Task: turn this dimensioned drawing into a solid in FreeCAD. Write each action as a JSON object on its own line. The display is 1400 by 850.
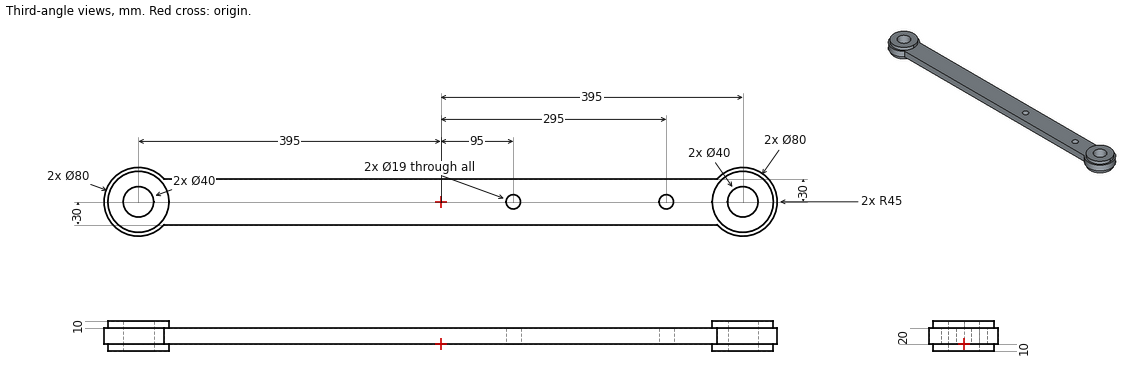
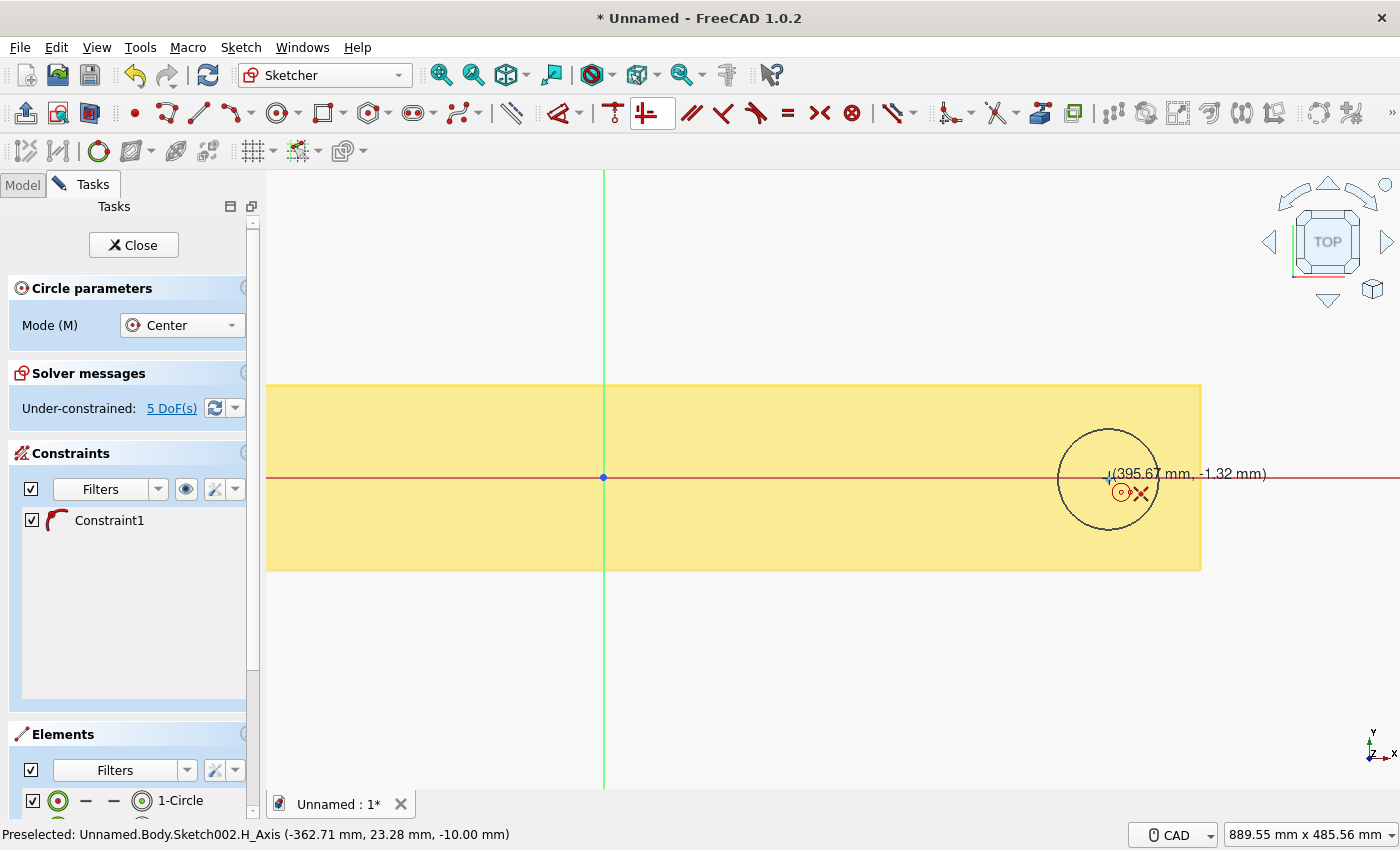
{"action": "left_click", "coordinate": [1108, 479]}
{"action": "left_click", "coordinate": [1126, 460]}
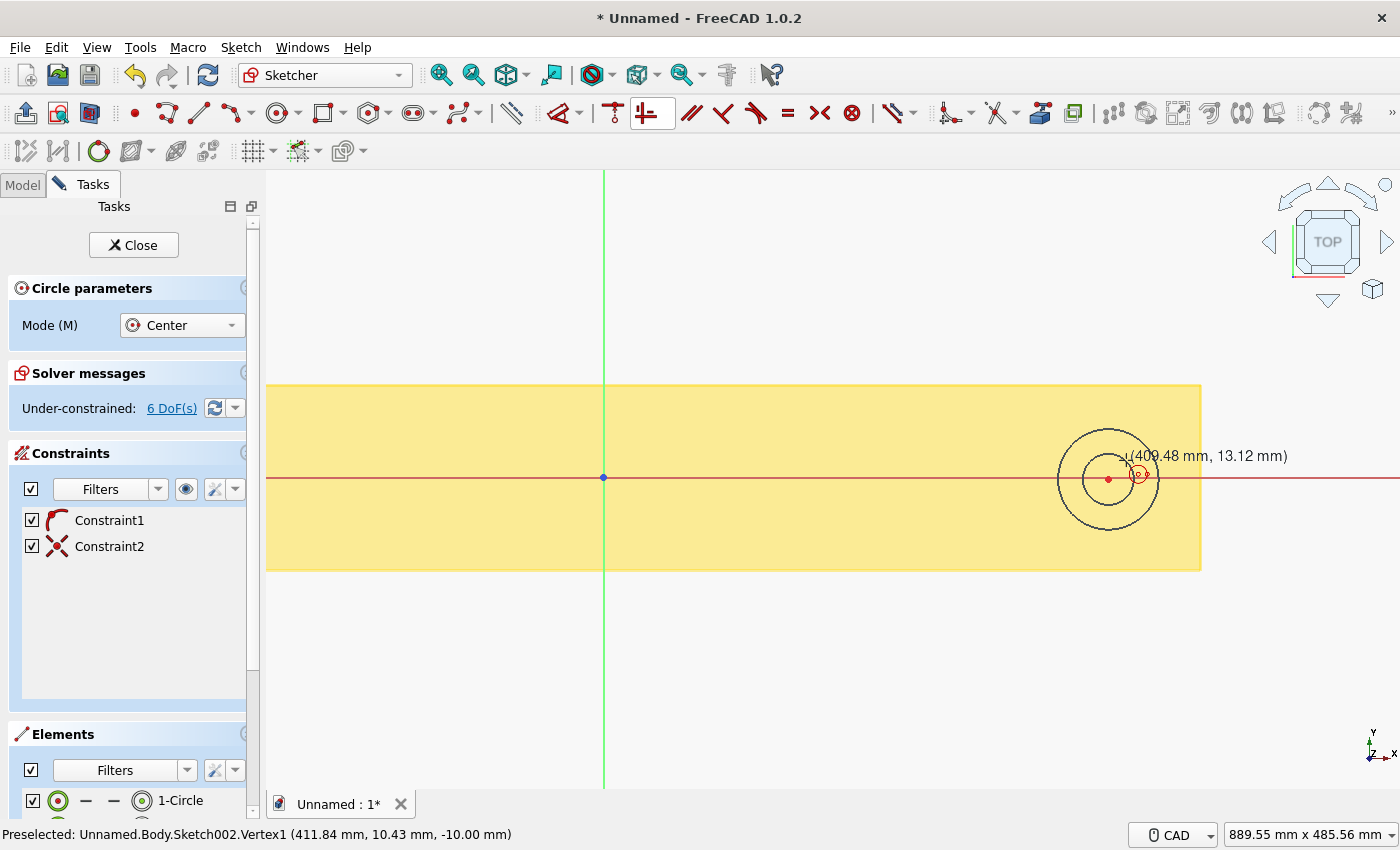
{"action": "scroll", "coordinate": [960, 482], "scroll_direction": "down", "scroll_amount": 3}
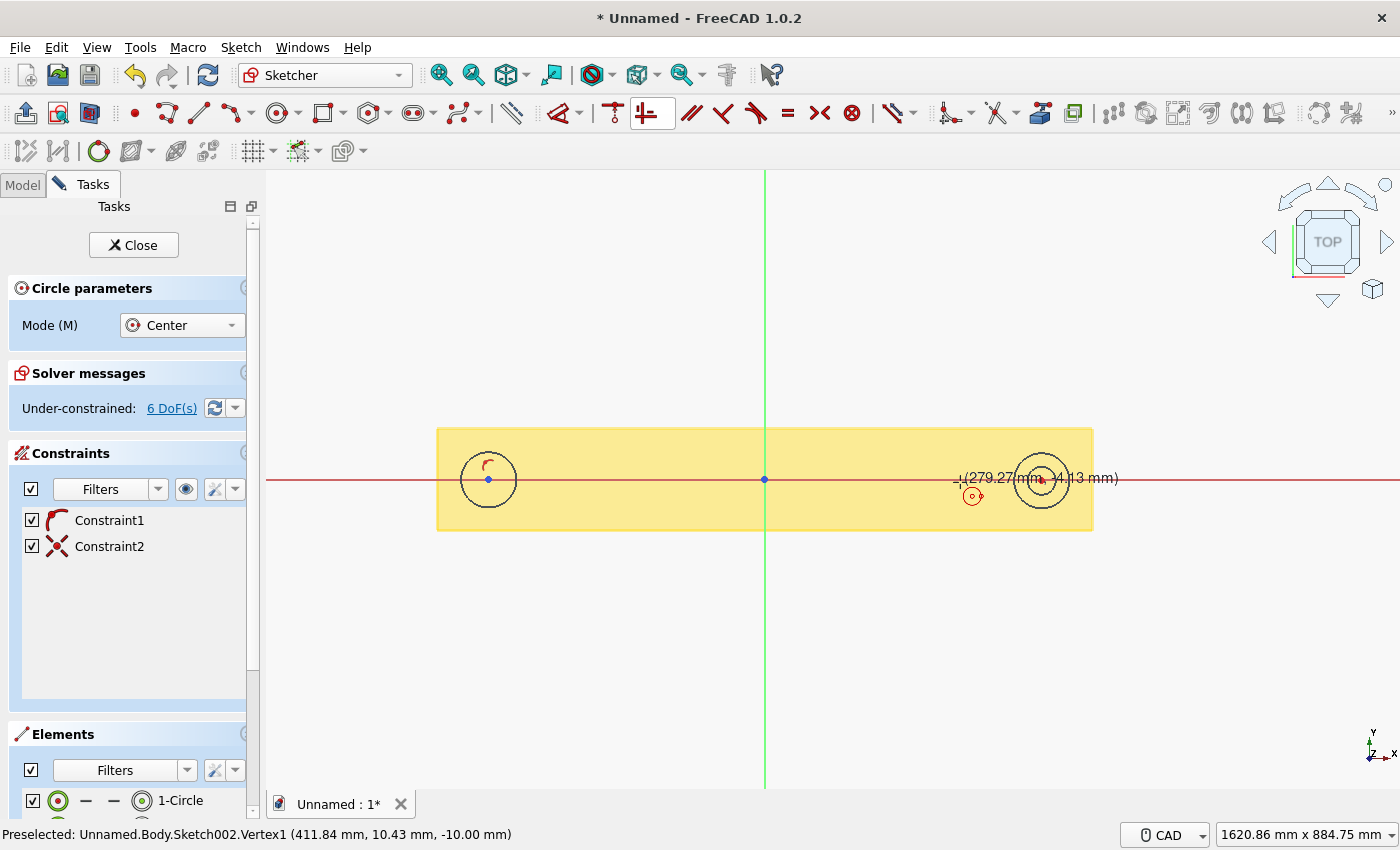
{"action": "scroll", "coordinate": [489, 480], "scroll_direction": "up", "scroll_amount": 3}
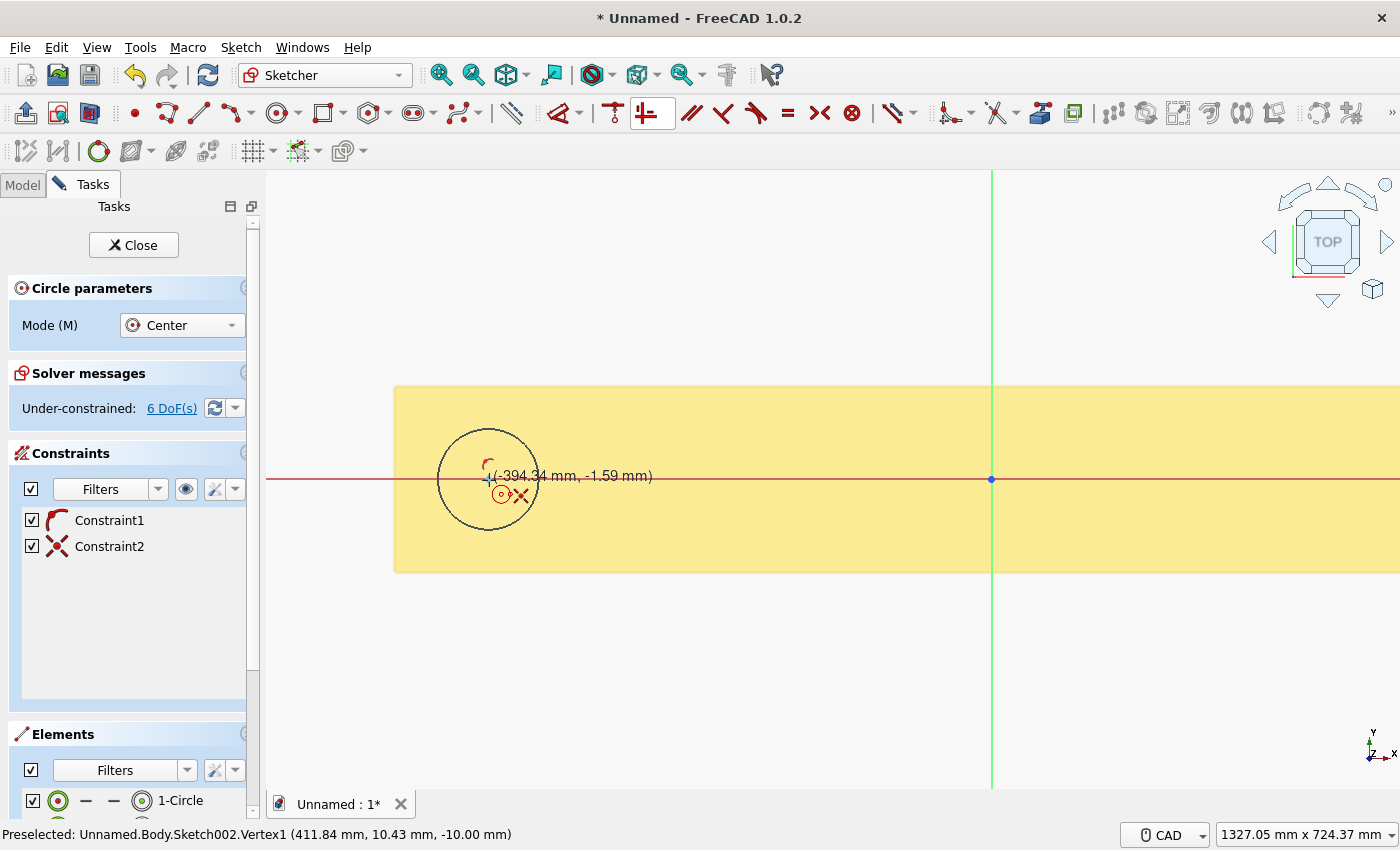
{"action": "left_click", "coordinate": [488, 479]}
{"action": "left_click", "coordinate": [506, 461]}
{"action": "key", "text": "Escape"}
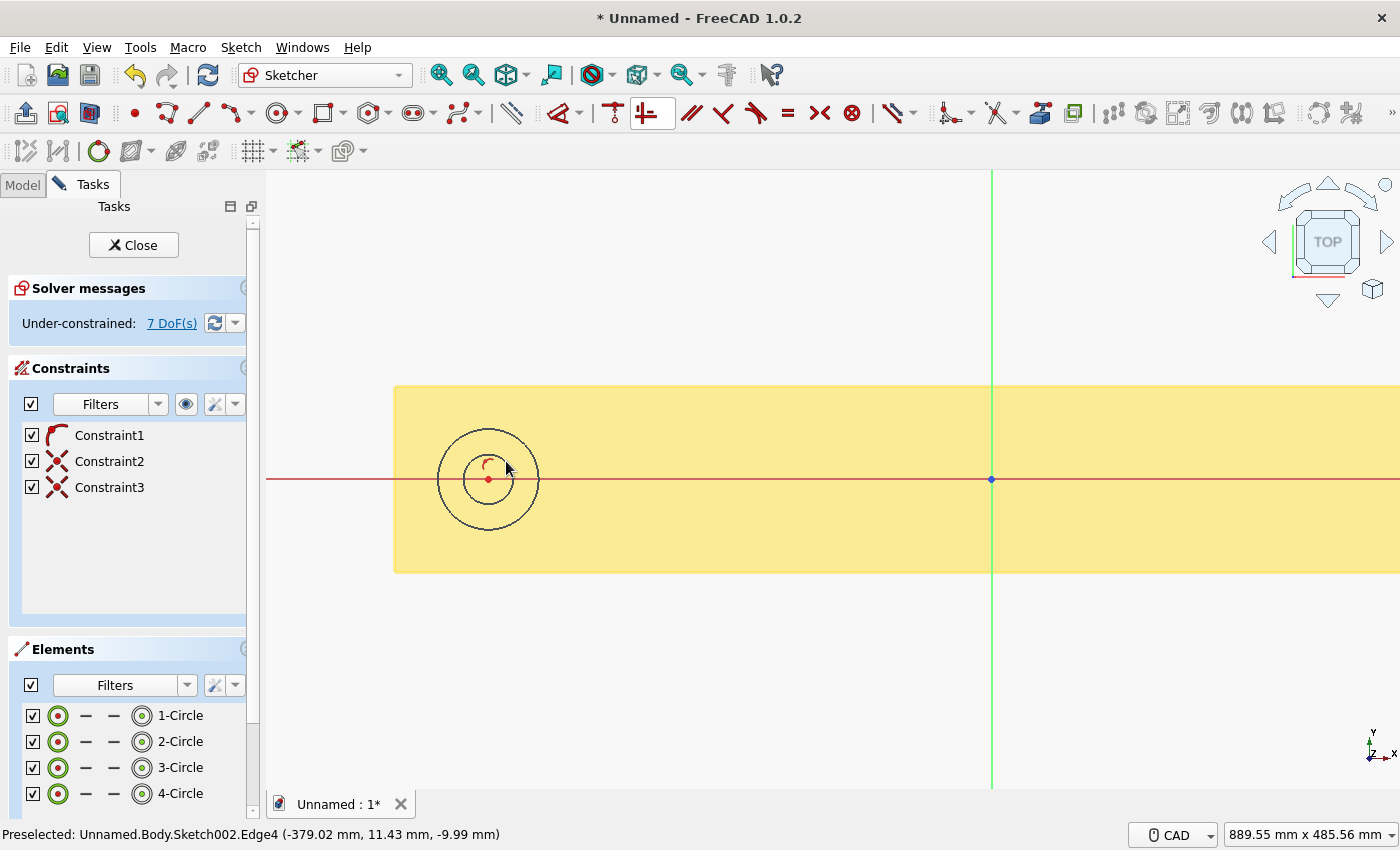
{"action": "scroll", "coordinate": [488, 480], "scroll_direction": "down", "scroll_amount": 3}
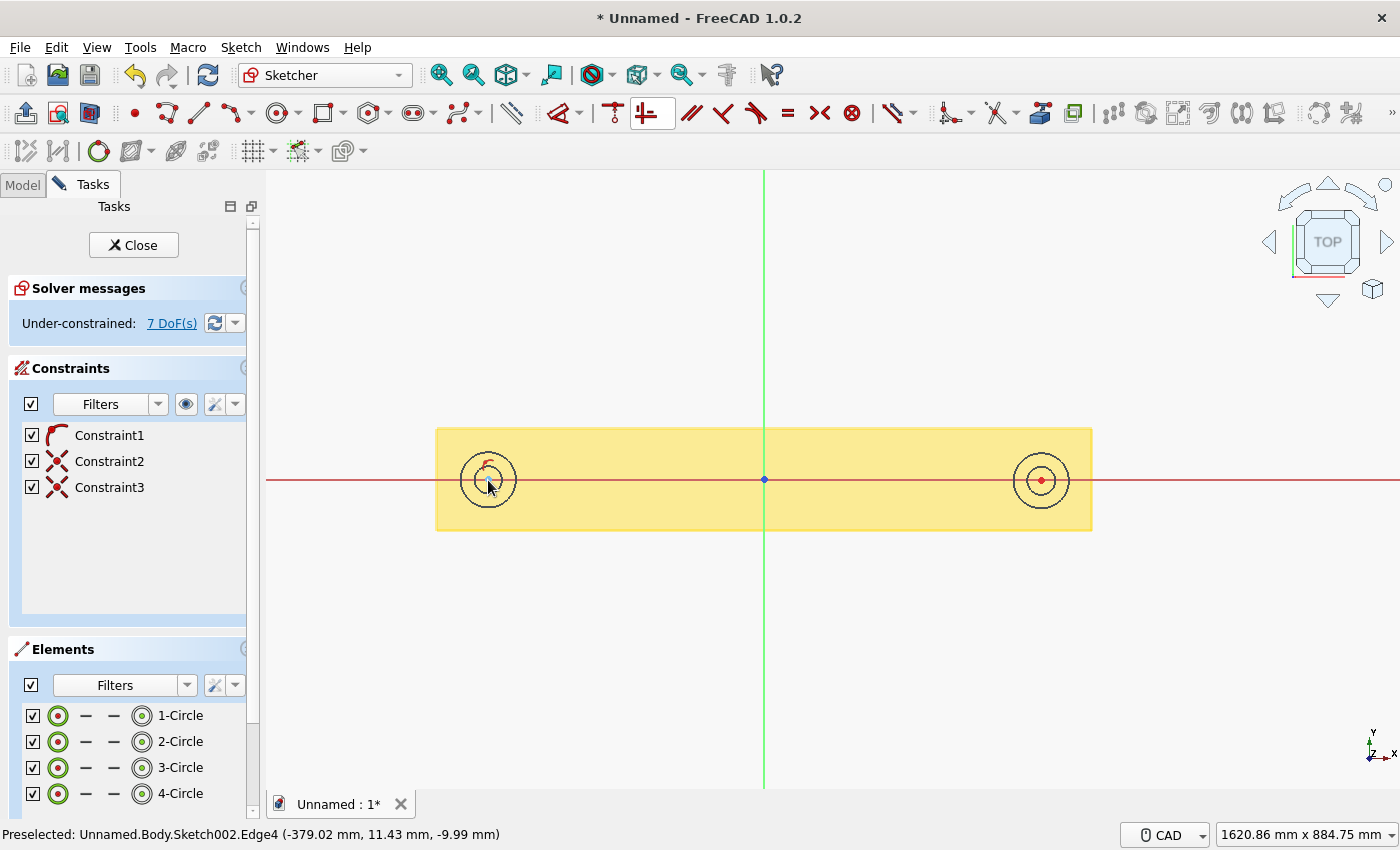
{"action": "left_click", "coordinate": [1061, 461]}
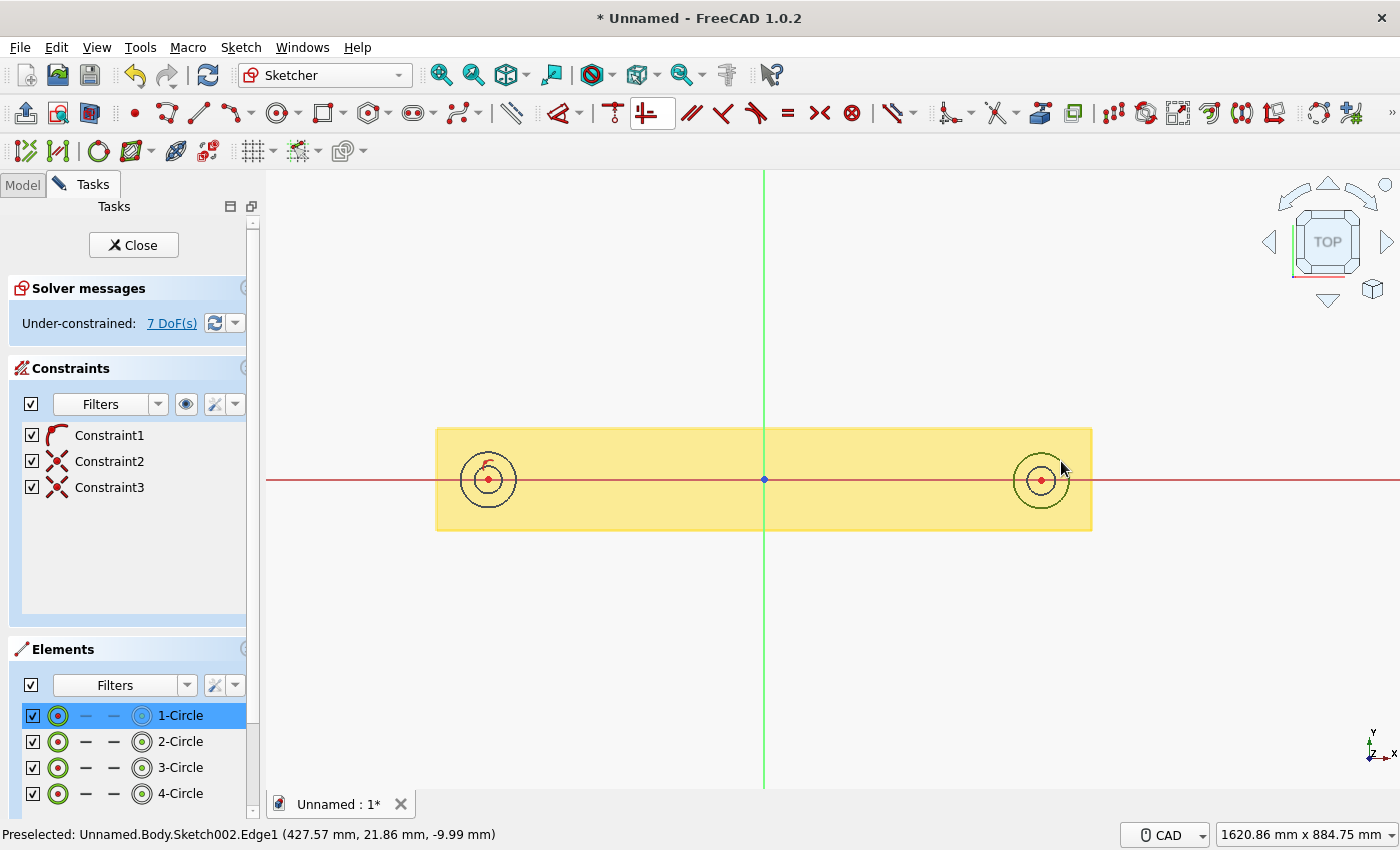
{"action": "left_click", "coordinate": [508, 460]}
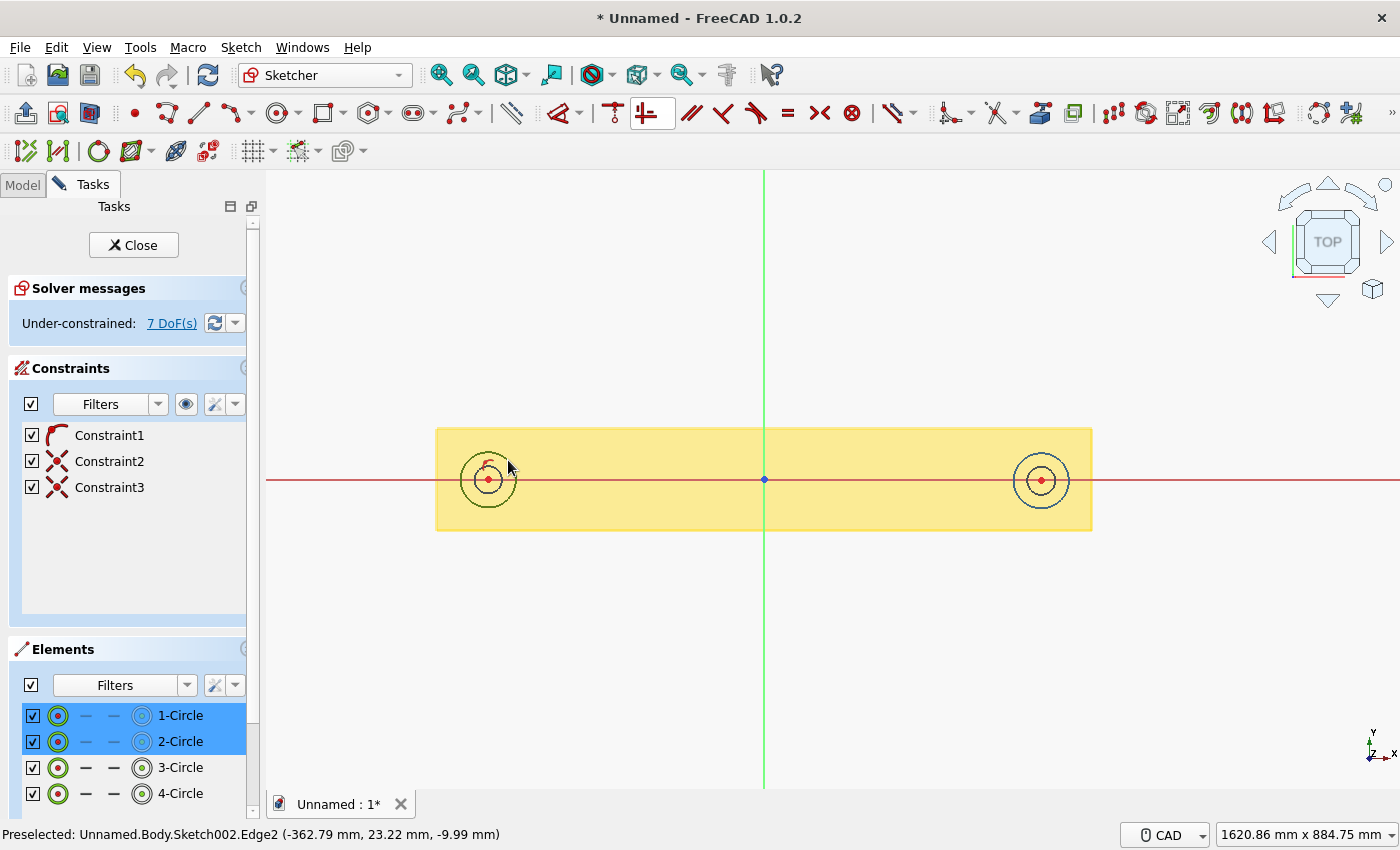
{"action": "key", "text": "e"}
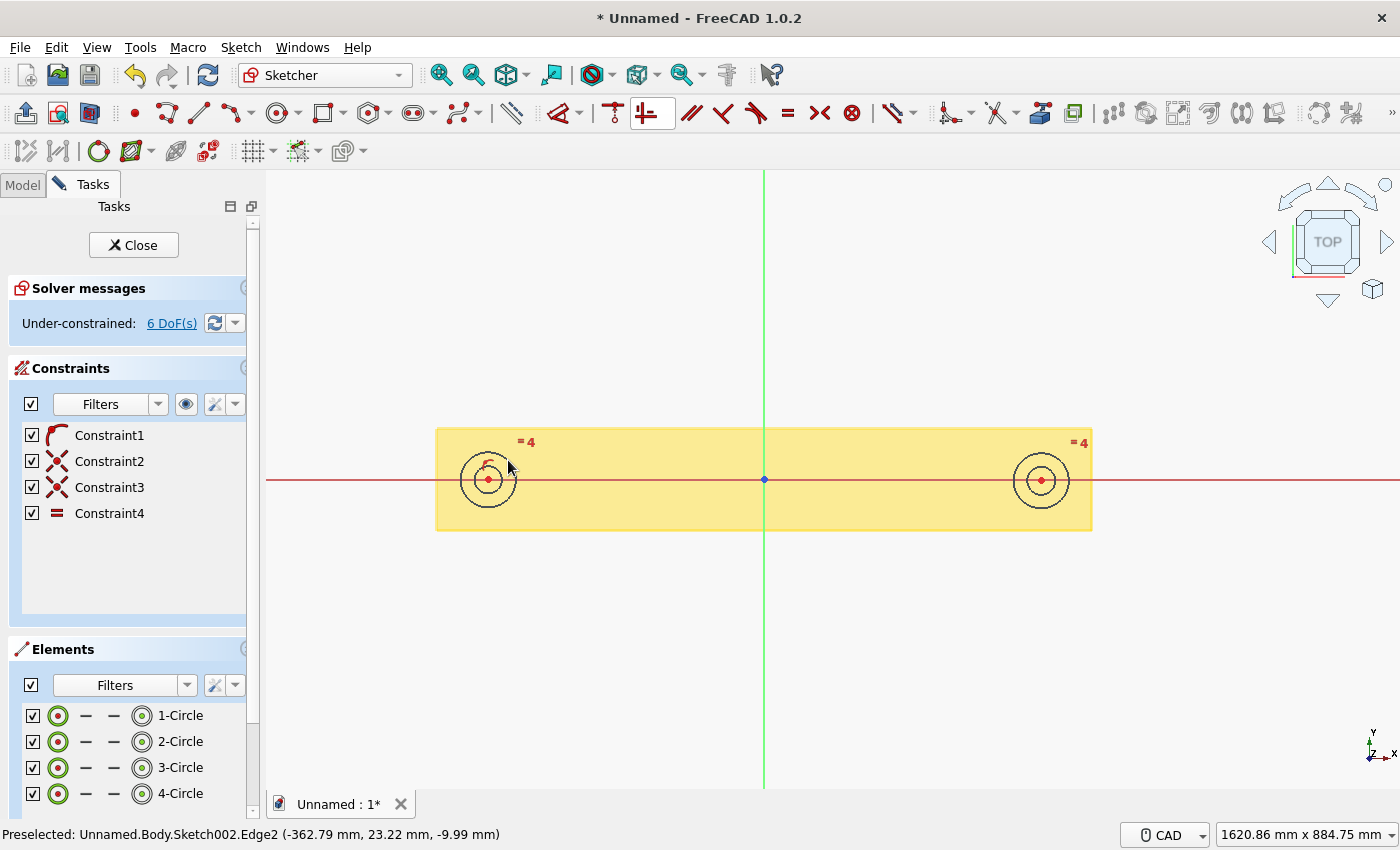
{"action": "scroll", "coordinate": [1031, 491], "scroll_direction": "up", "scroll_amount": 2}